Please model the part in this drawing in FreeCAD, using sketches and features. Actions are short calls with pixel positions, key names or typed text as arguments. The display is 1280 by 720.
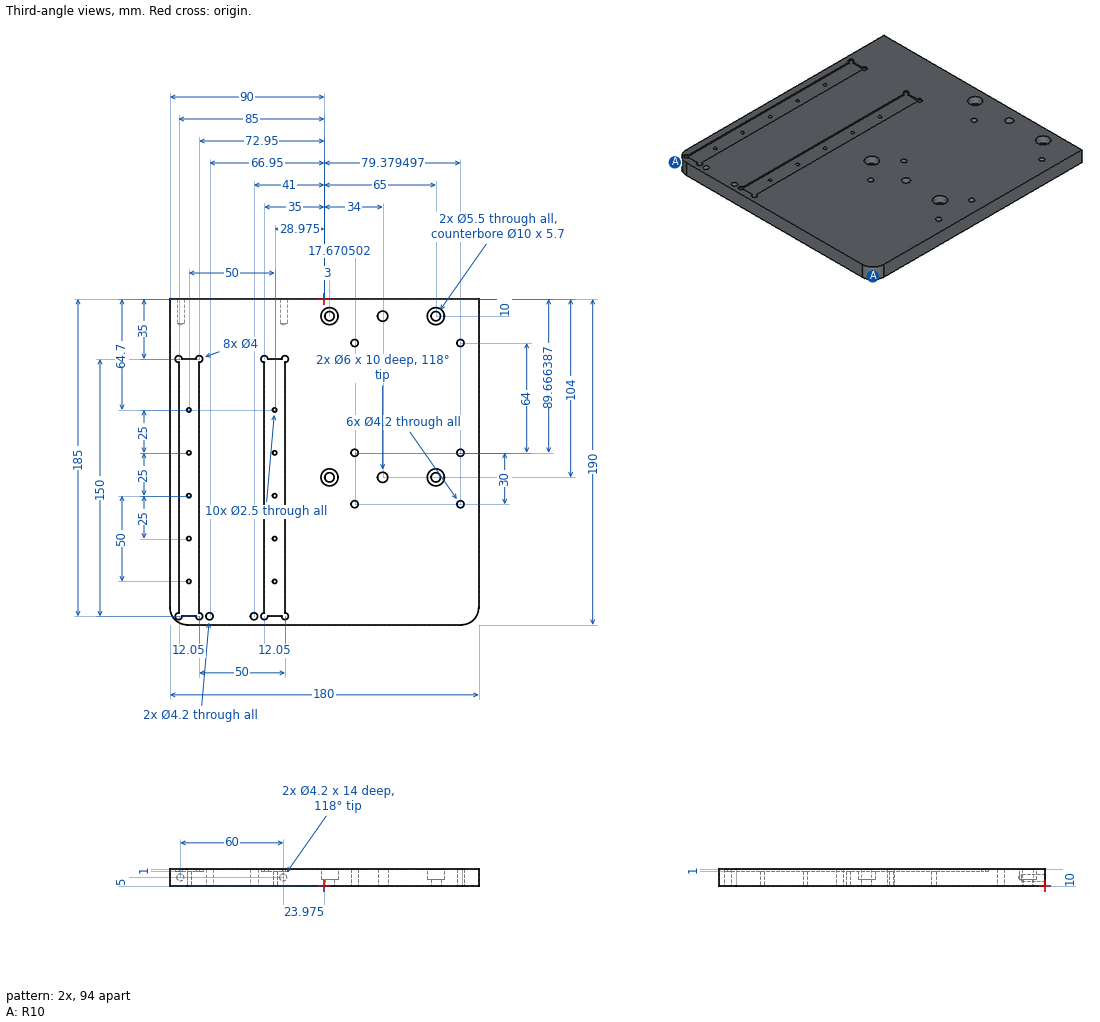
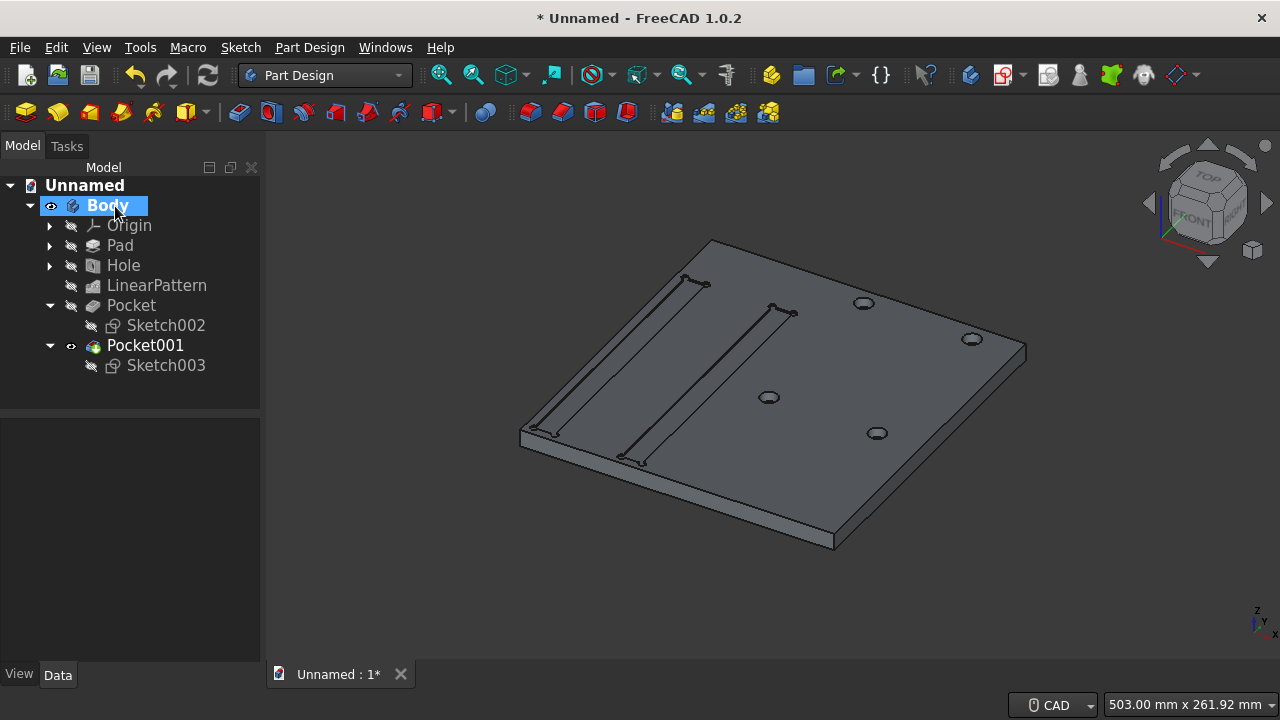
click(1004, 76)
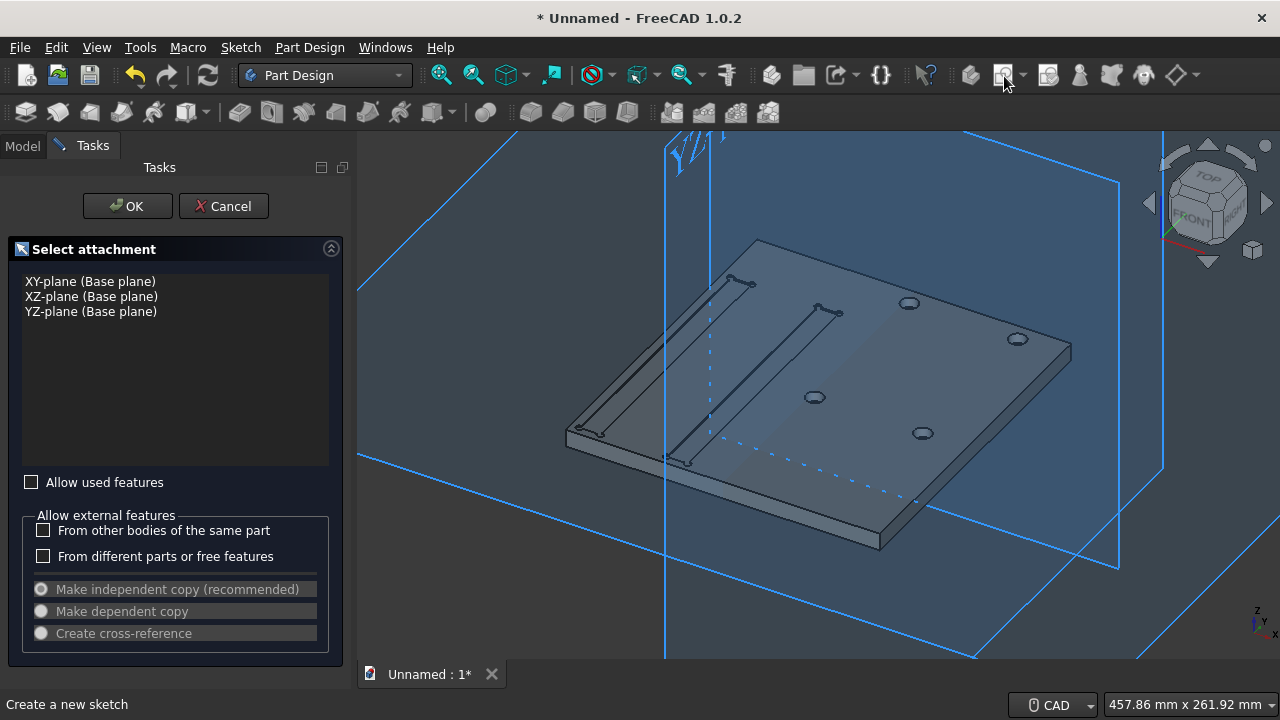
click(82, 296)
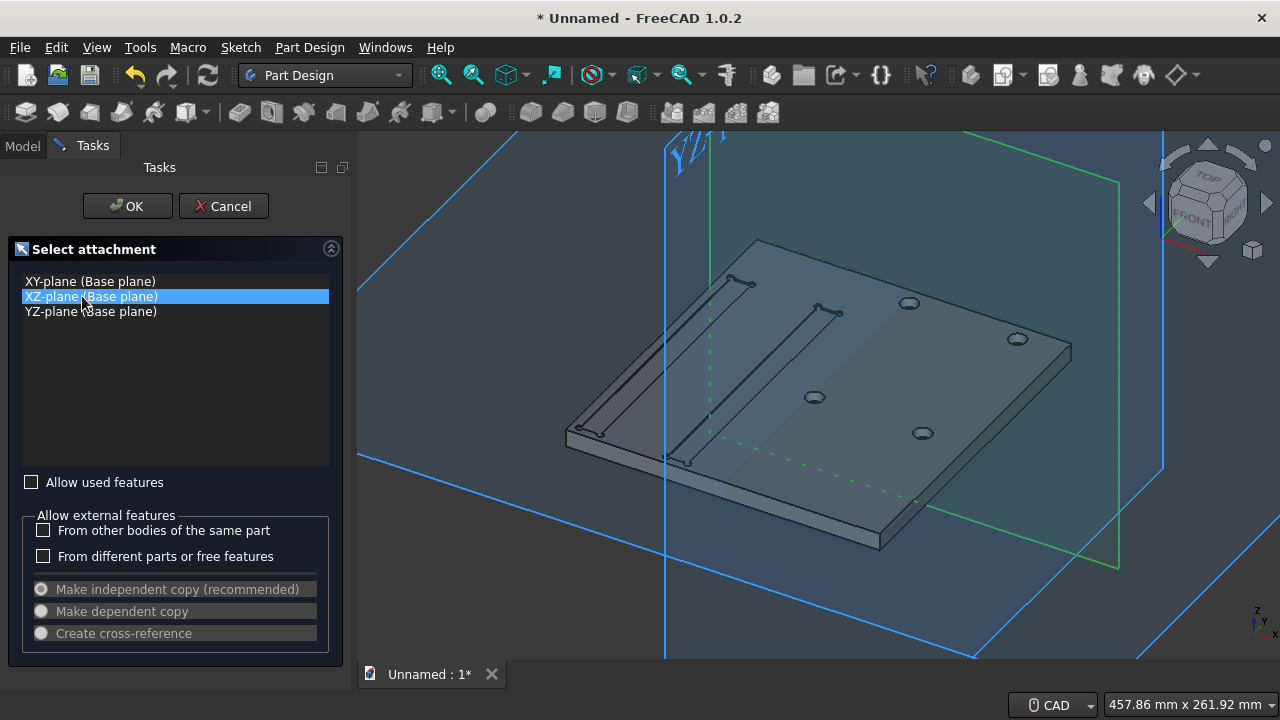
click(128, 206)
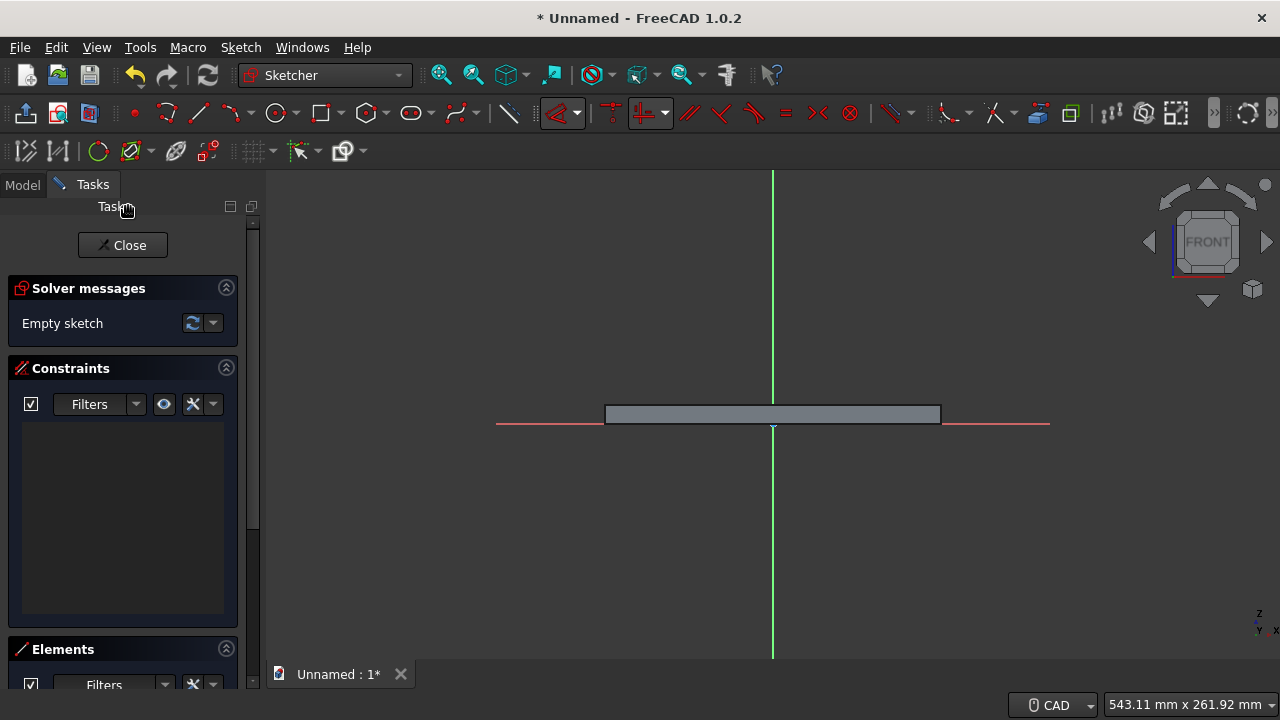
click(90, 114)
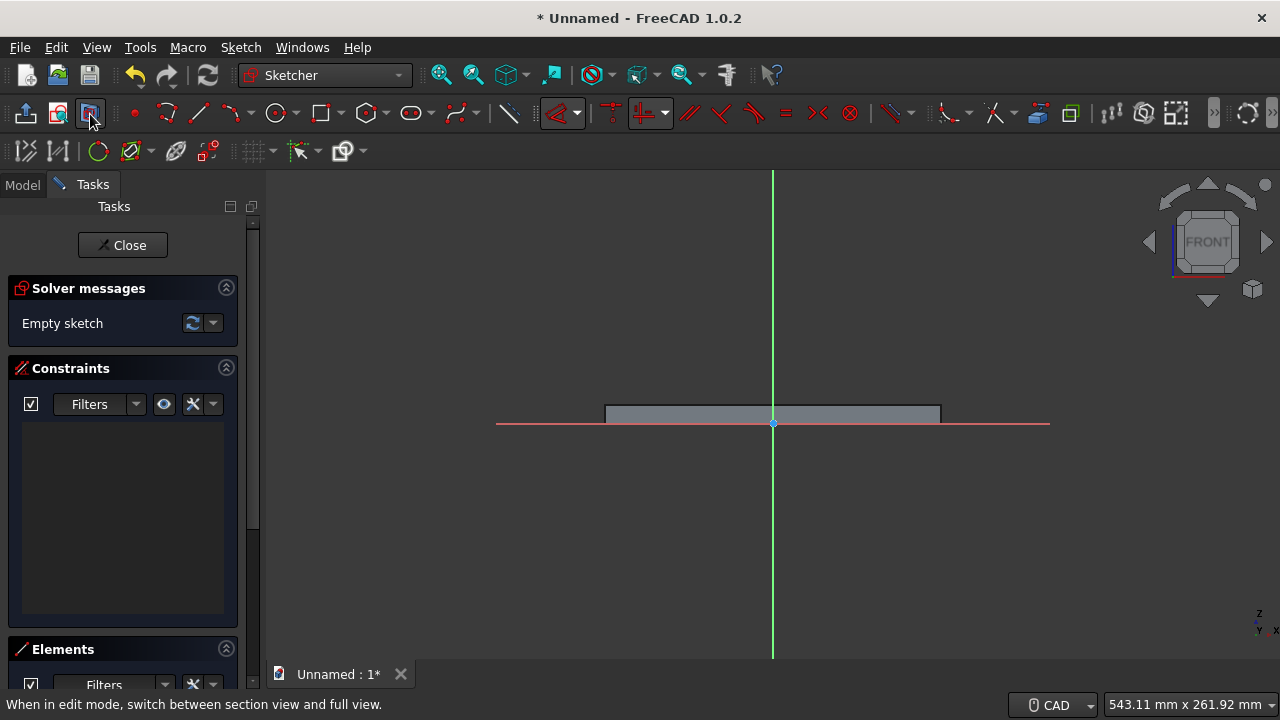
scroll(688, 418, up, 6)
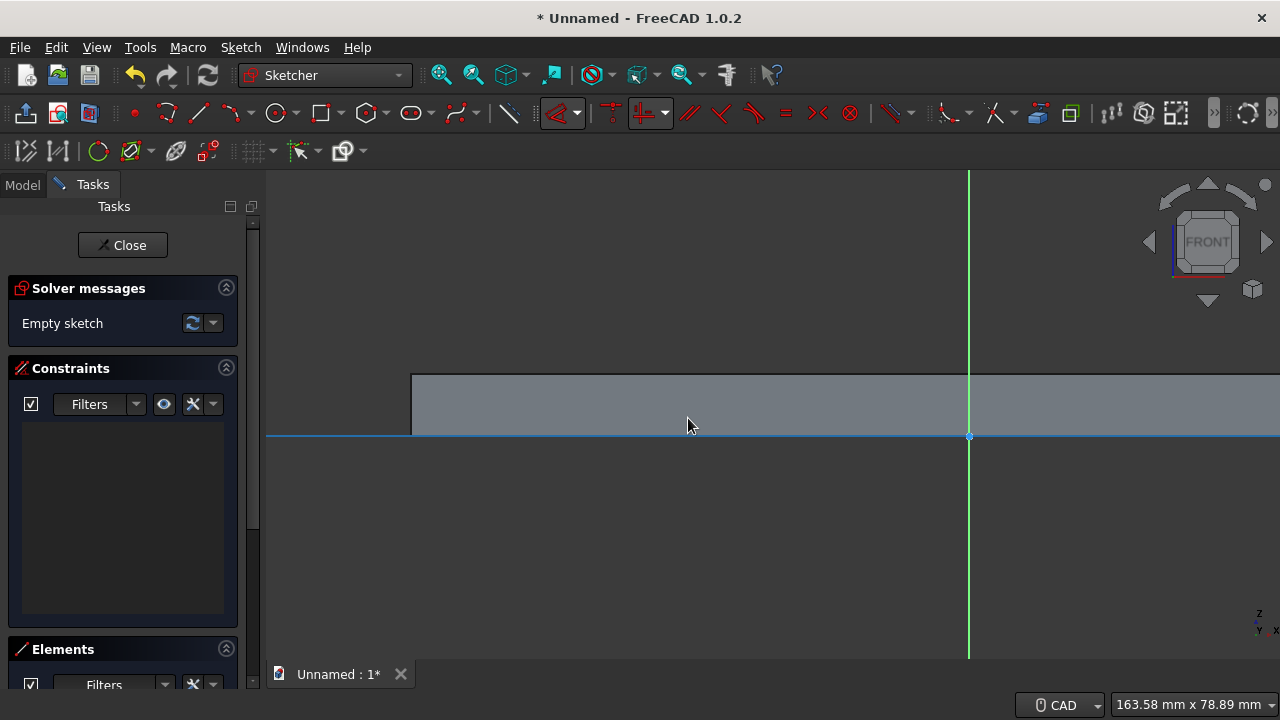
key(g)
key(c)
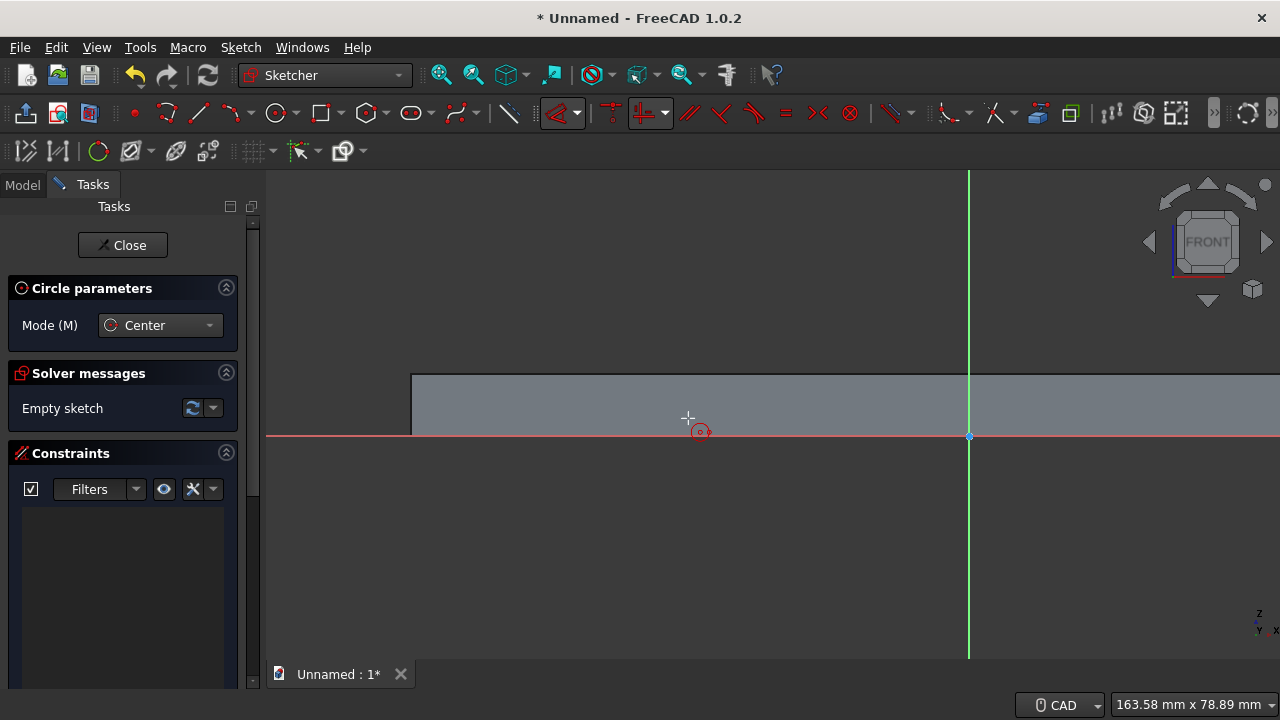
scroll(821, 405, up, 3)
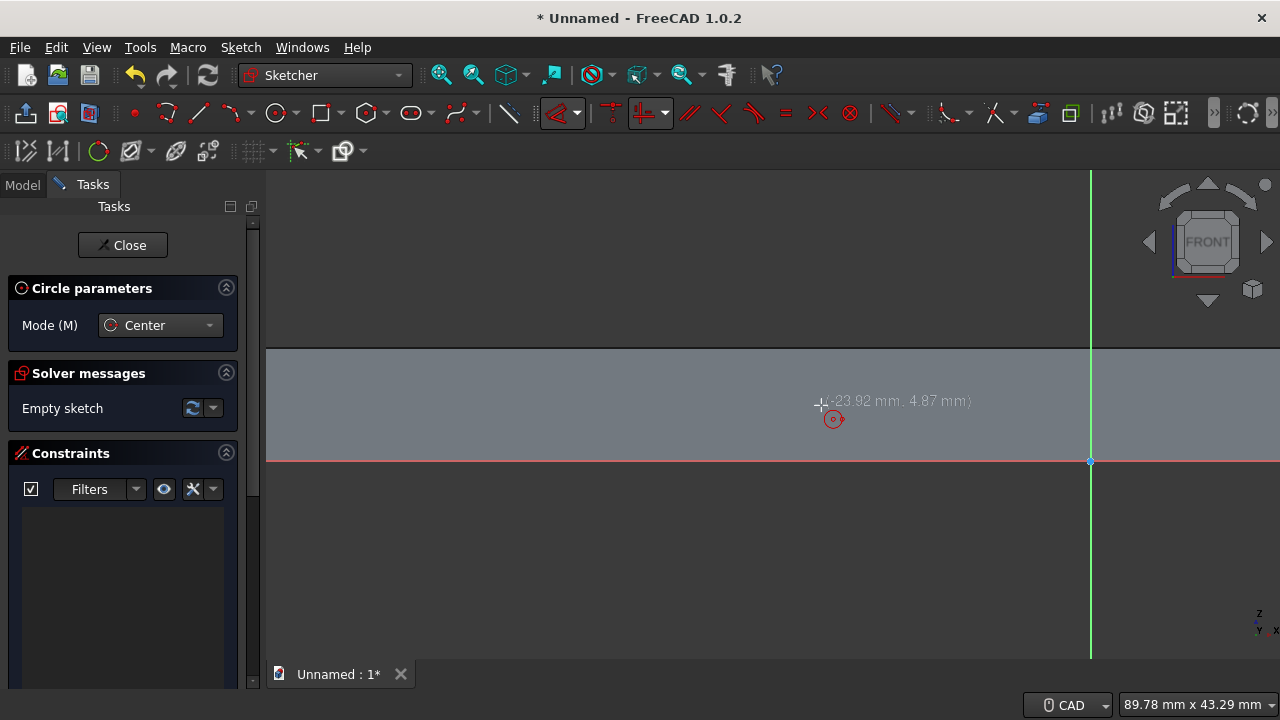
click(820, 405)
move(837, 388)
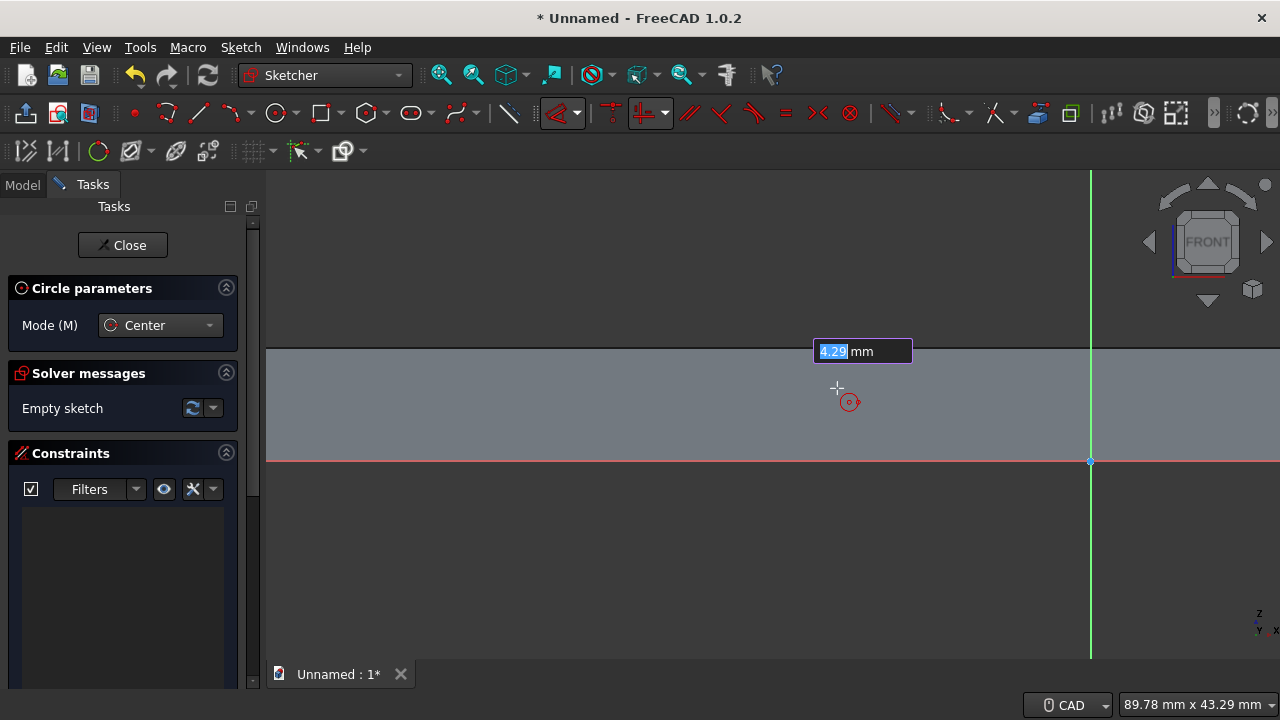
text(4.2)
key(Return)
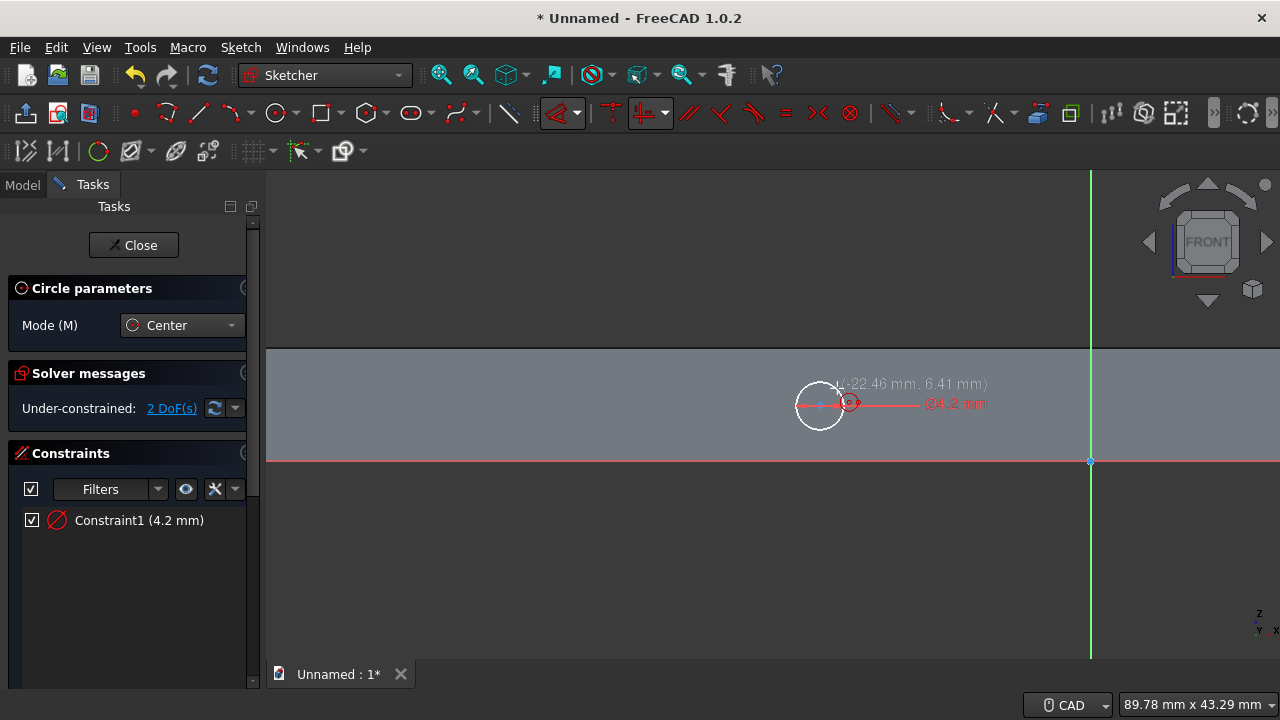
scroll(826, 406, down, 3)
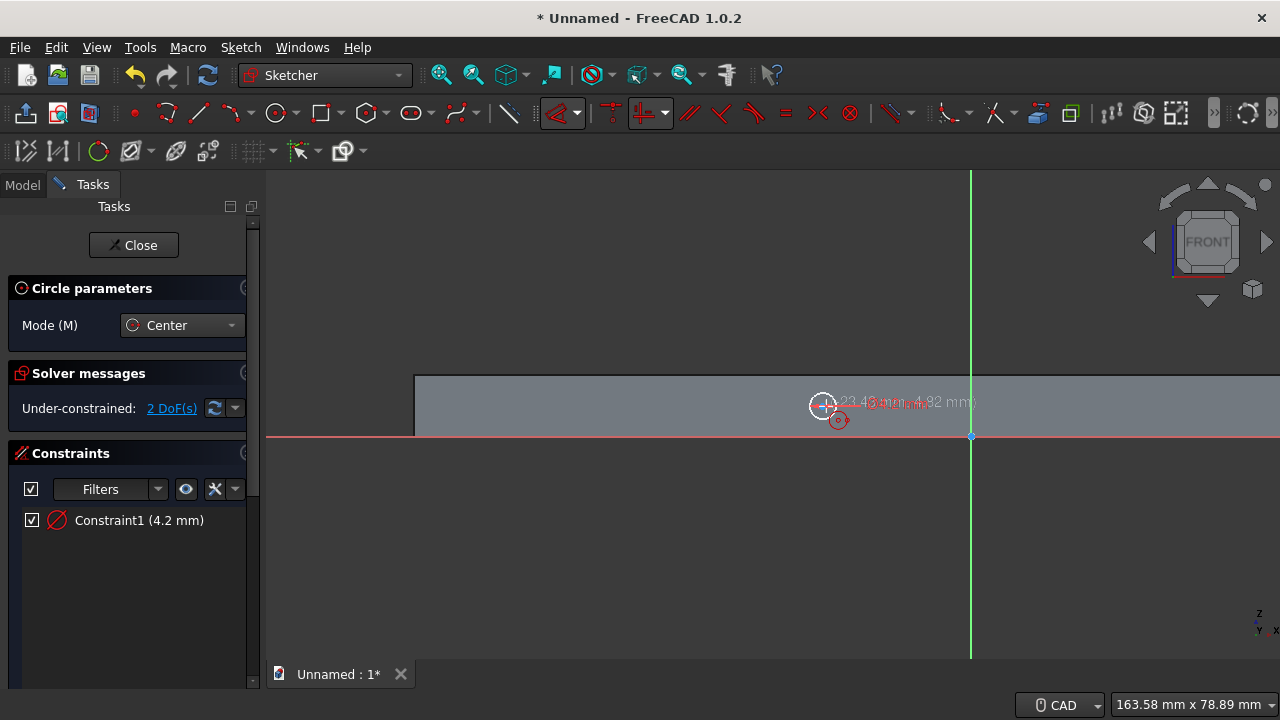
scroll(451, 406, up, 3)